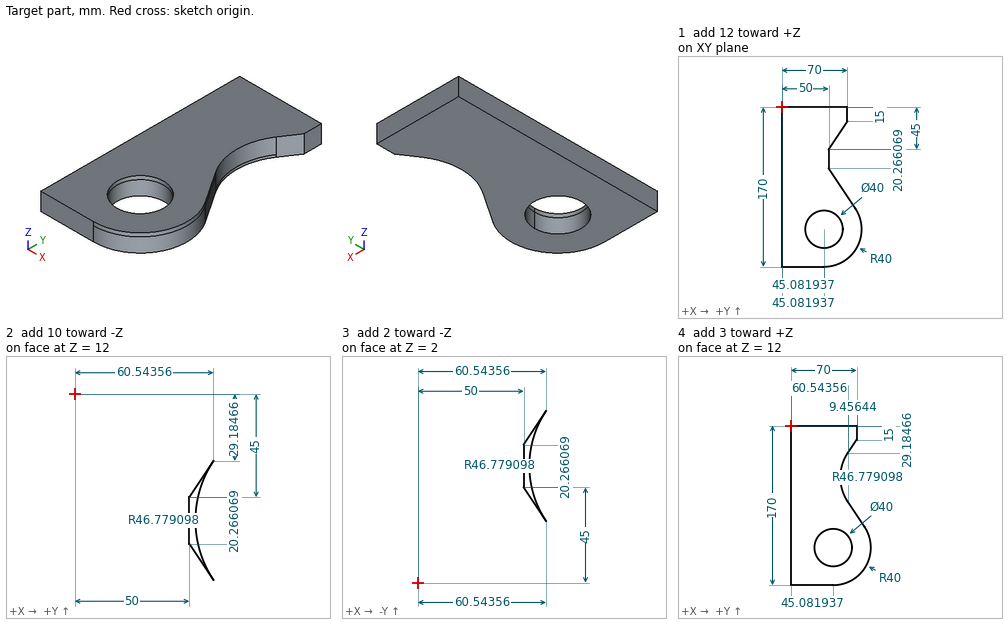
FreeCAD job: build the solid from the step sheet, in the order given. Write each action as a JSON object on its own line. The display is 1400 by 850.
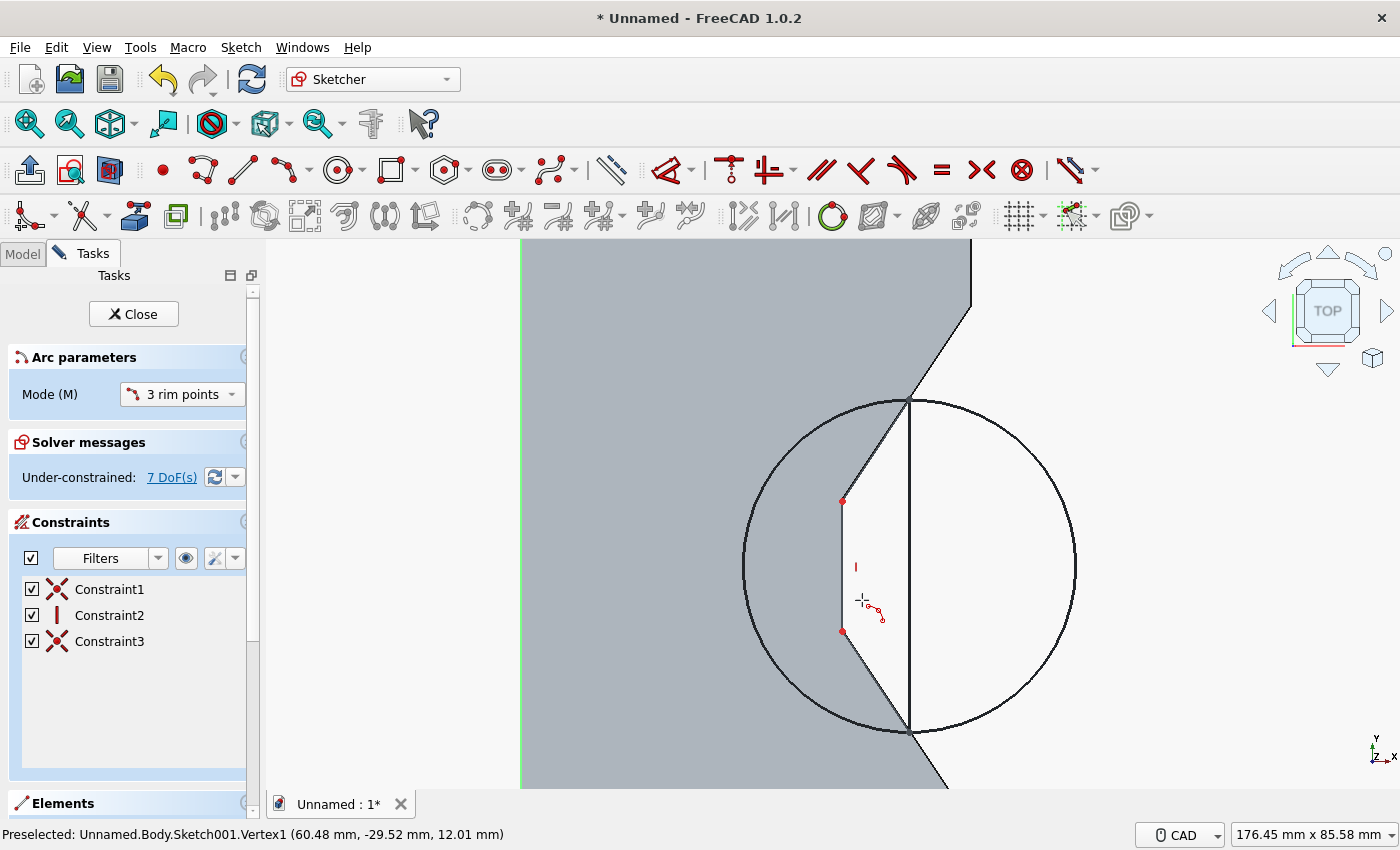
{"action": "left_click", "coordinate": [861, 600]}
{"action": "key", "text": "Escape"}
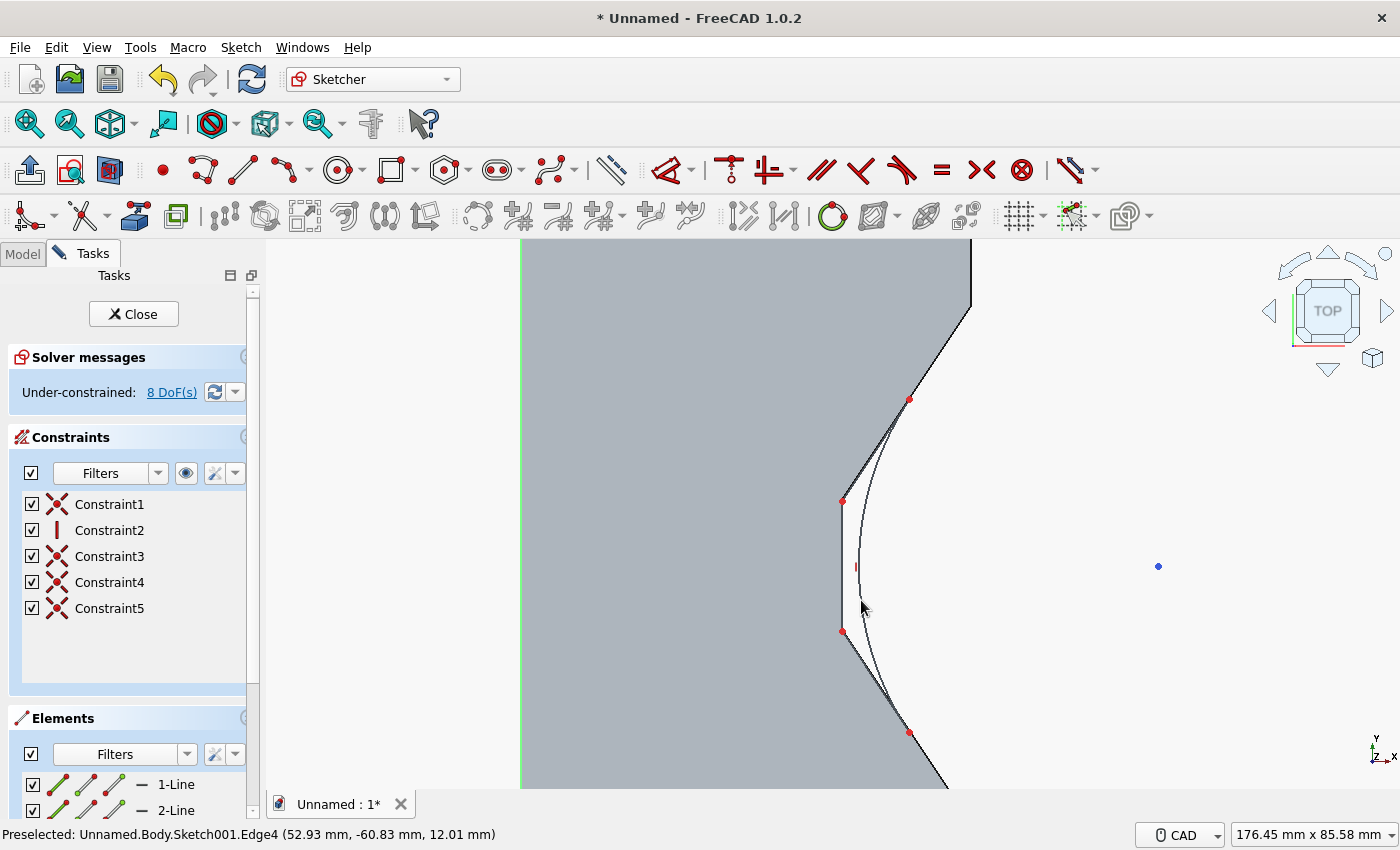
{"action": "left_click", "coordinate": [862, 471]}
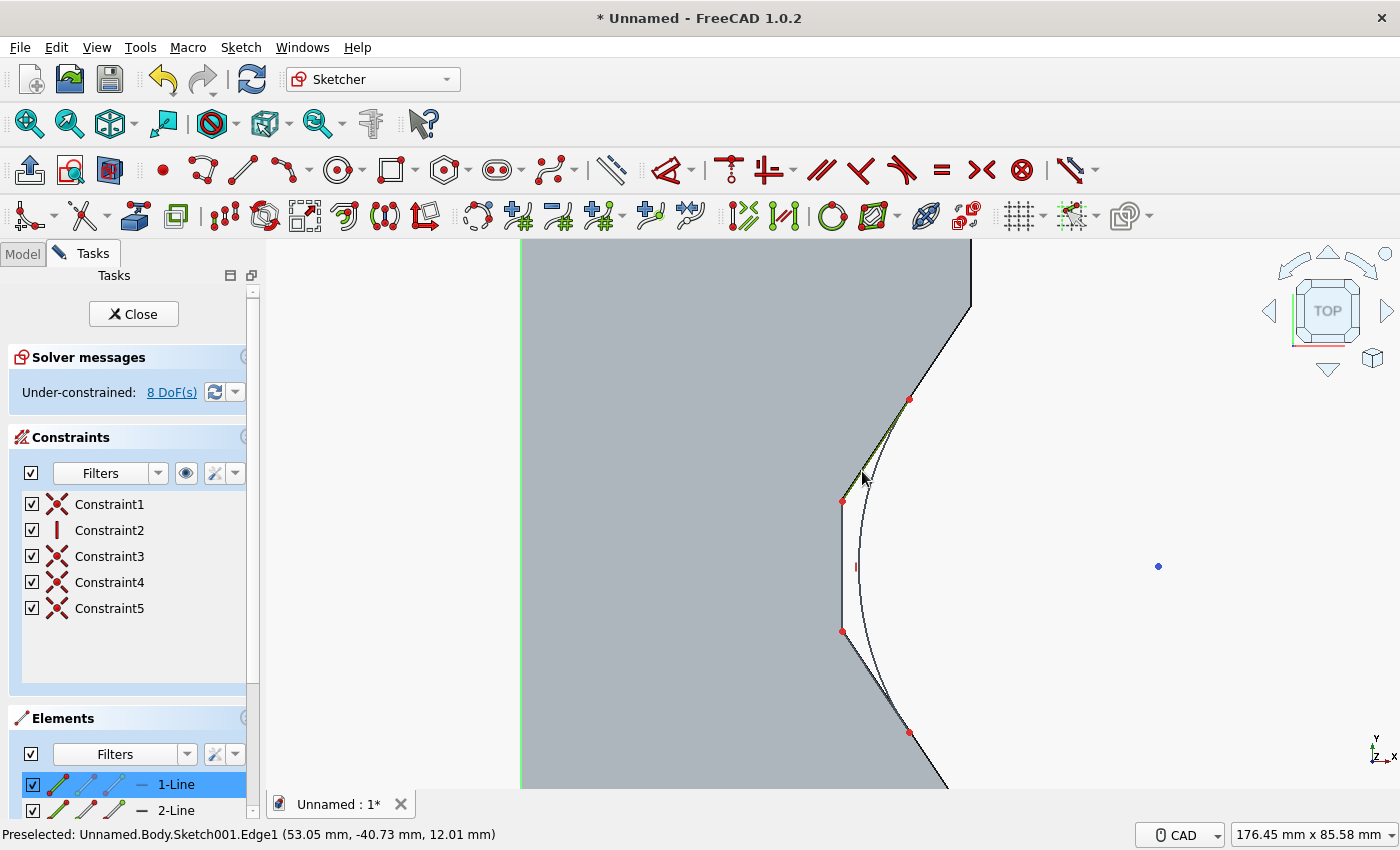
{"action": "left_click", "coordinate": [867, 496]}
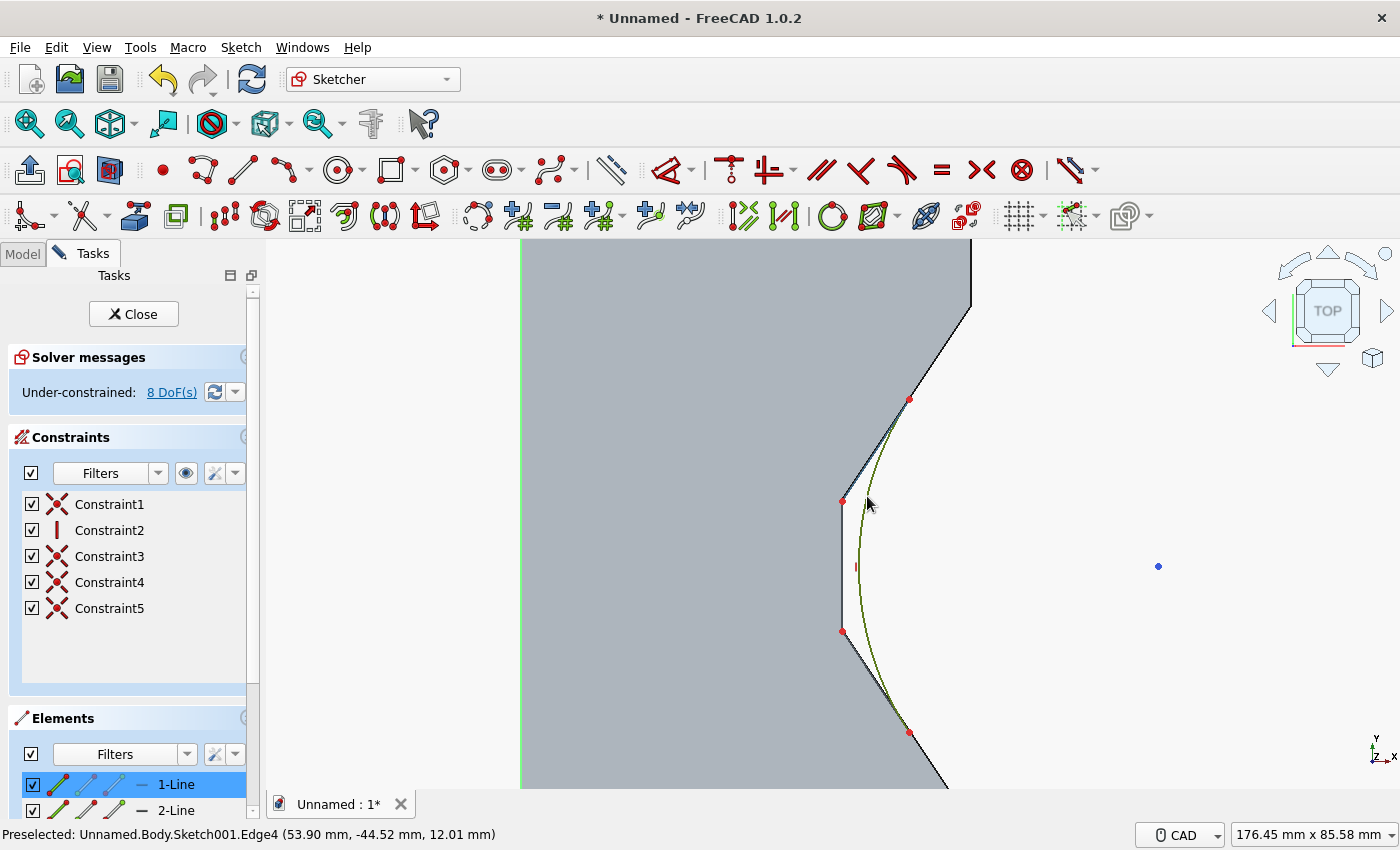
{"action": "left_click", "coordinate": [902, 170]}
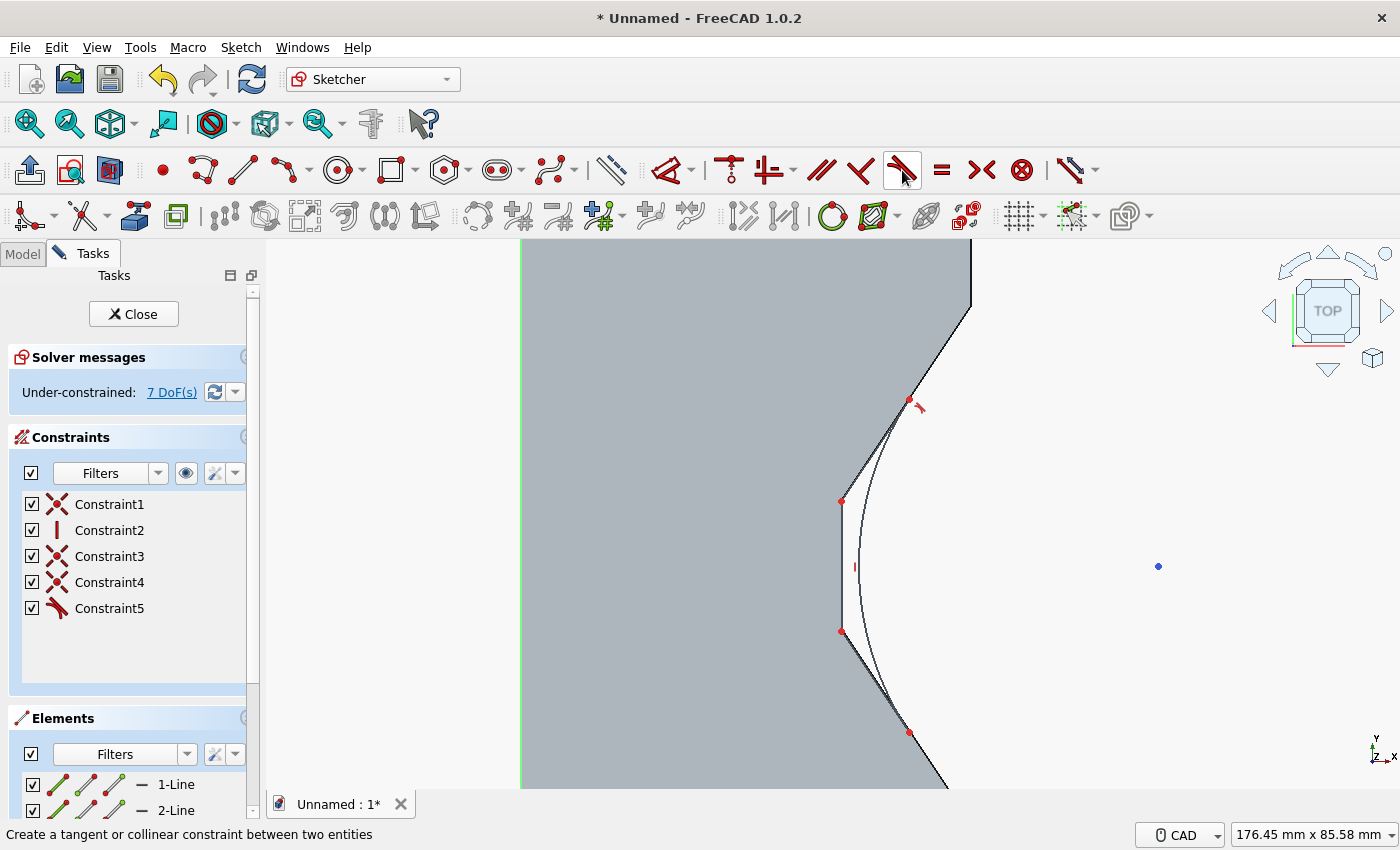
{"action": "left_click", "coordinate": [862, 661]}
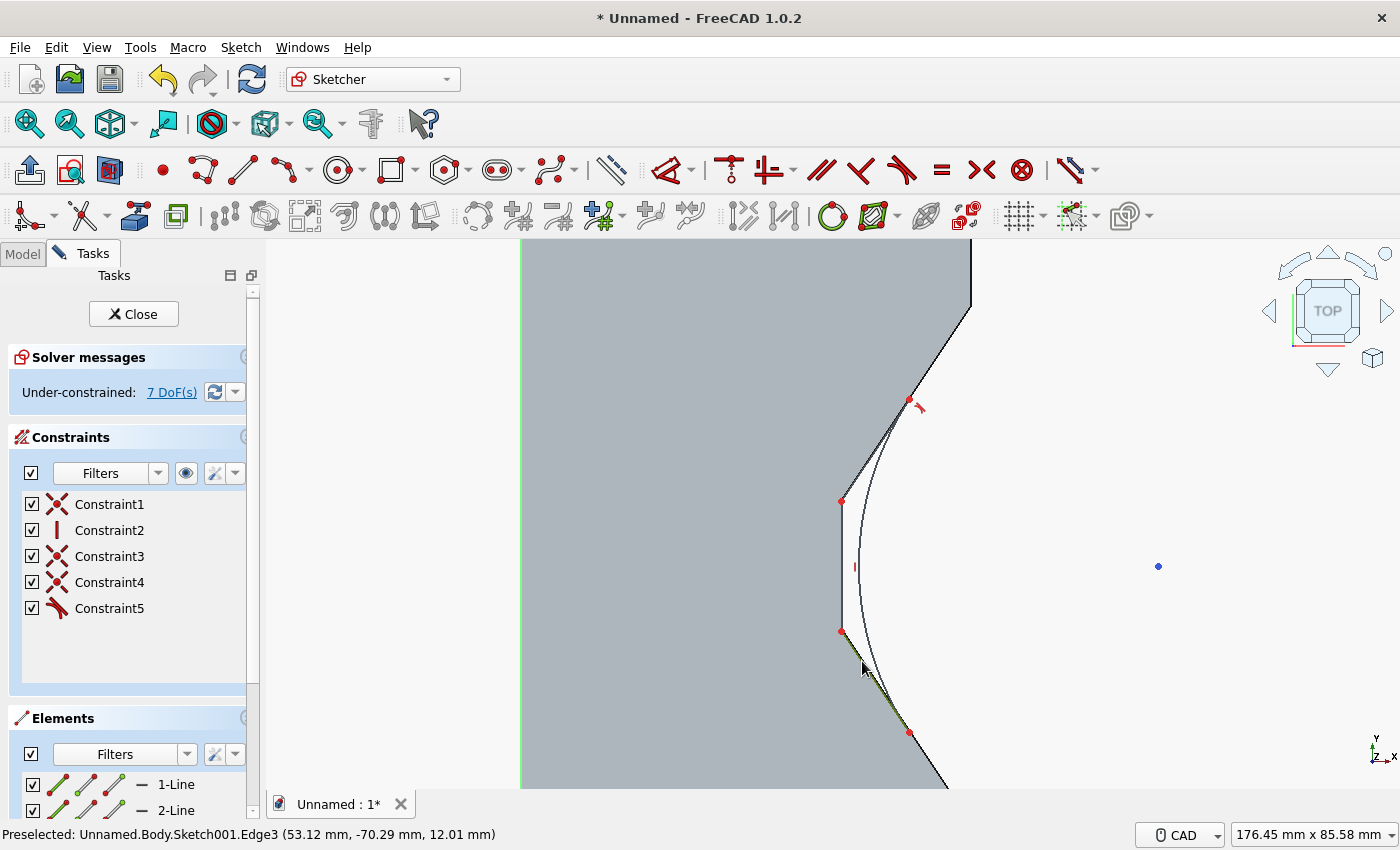
{"action": "left_click", "coordinate": [867, 496]}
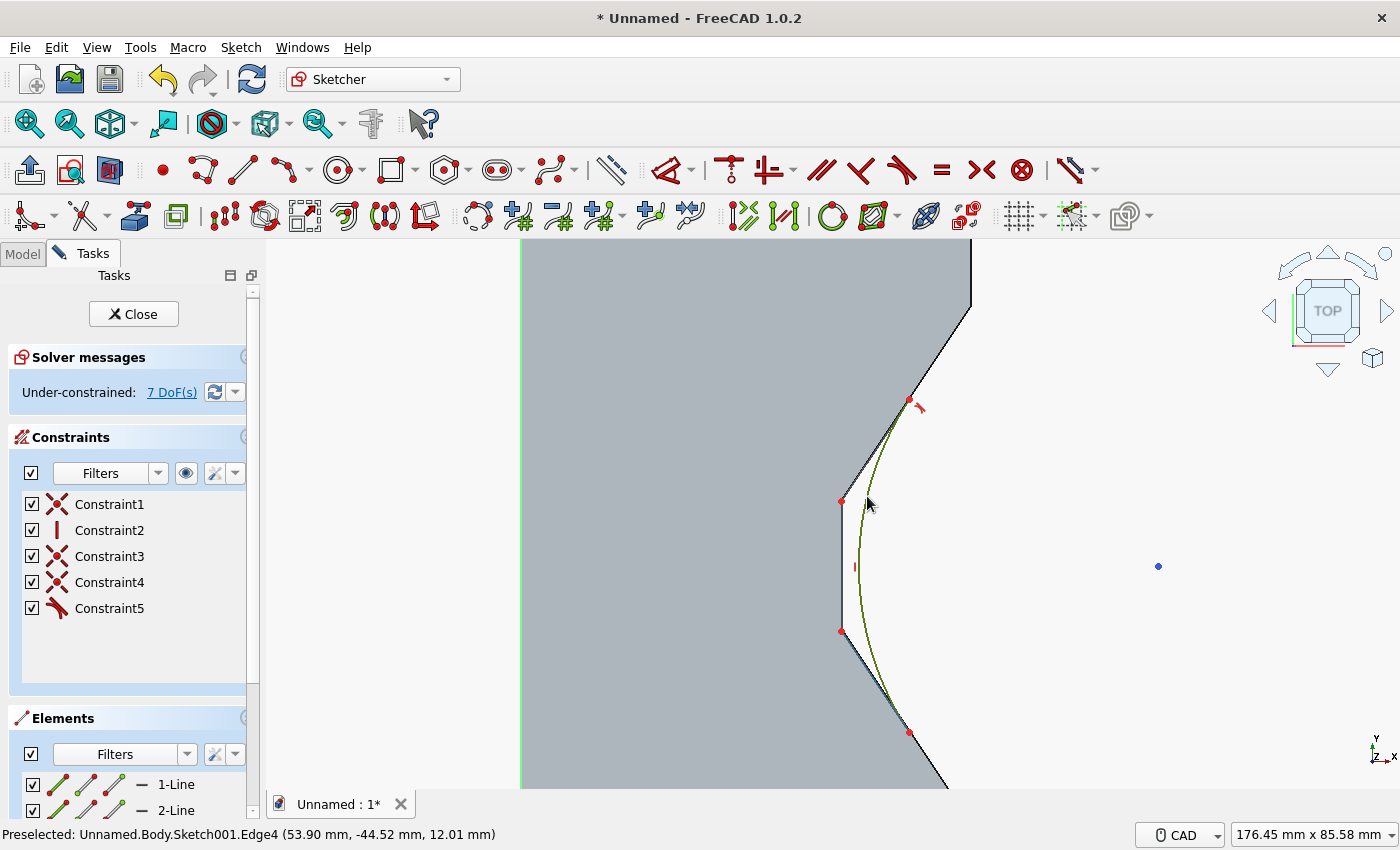
{"action": "left_click", "coordinate": [902, 170]}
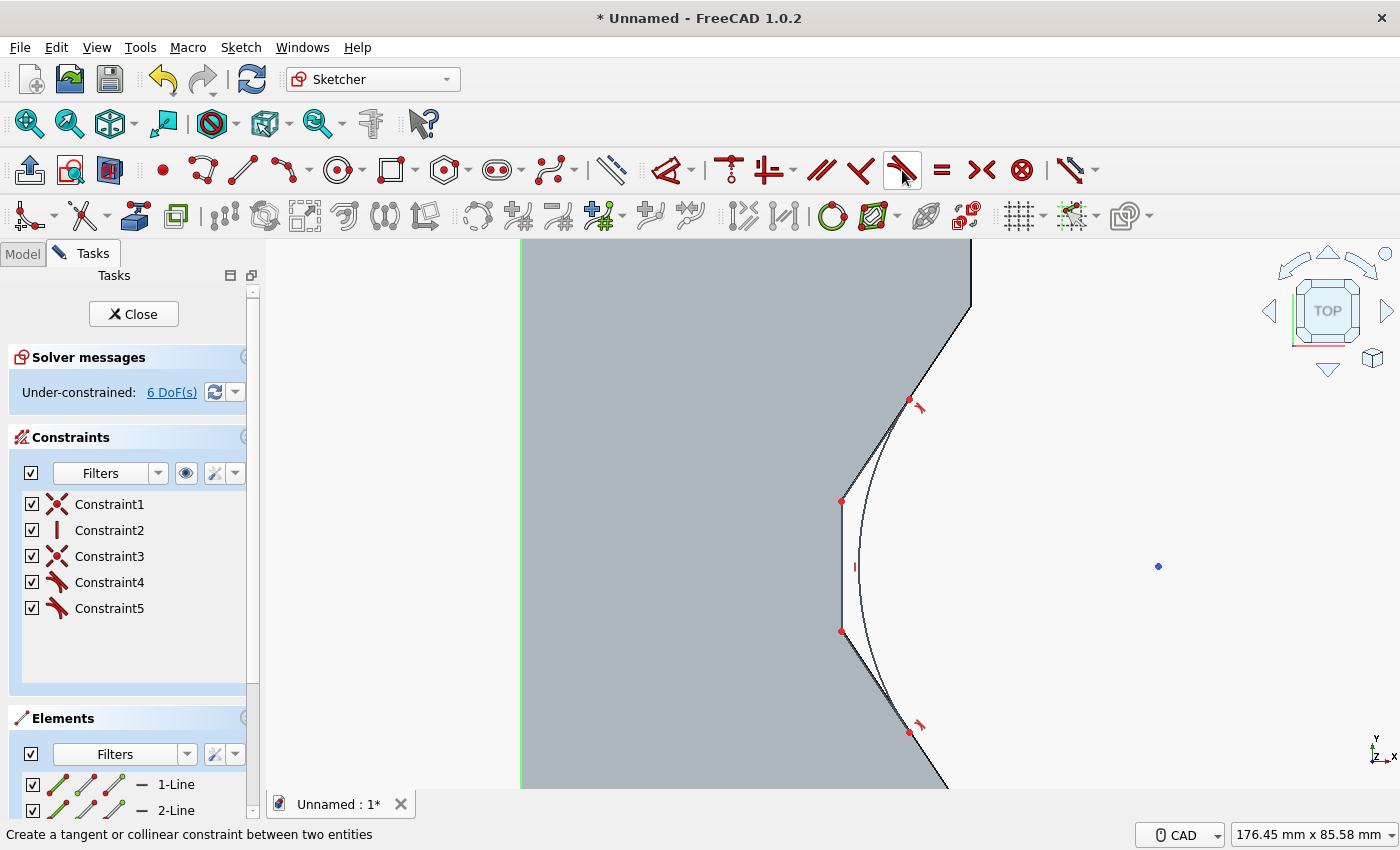
{"action": "left_click", "coordinate": [666, 170]}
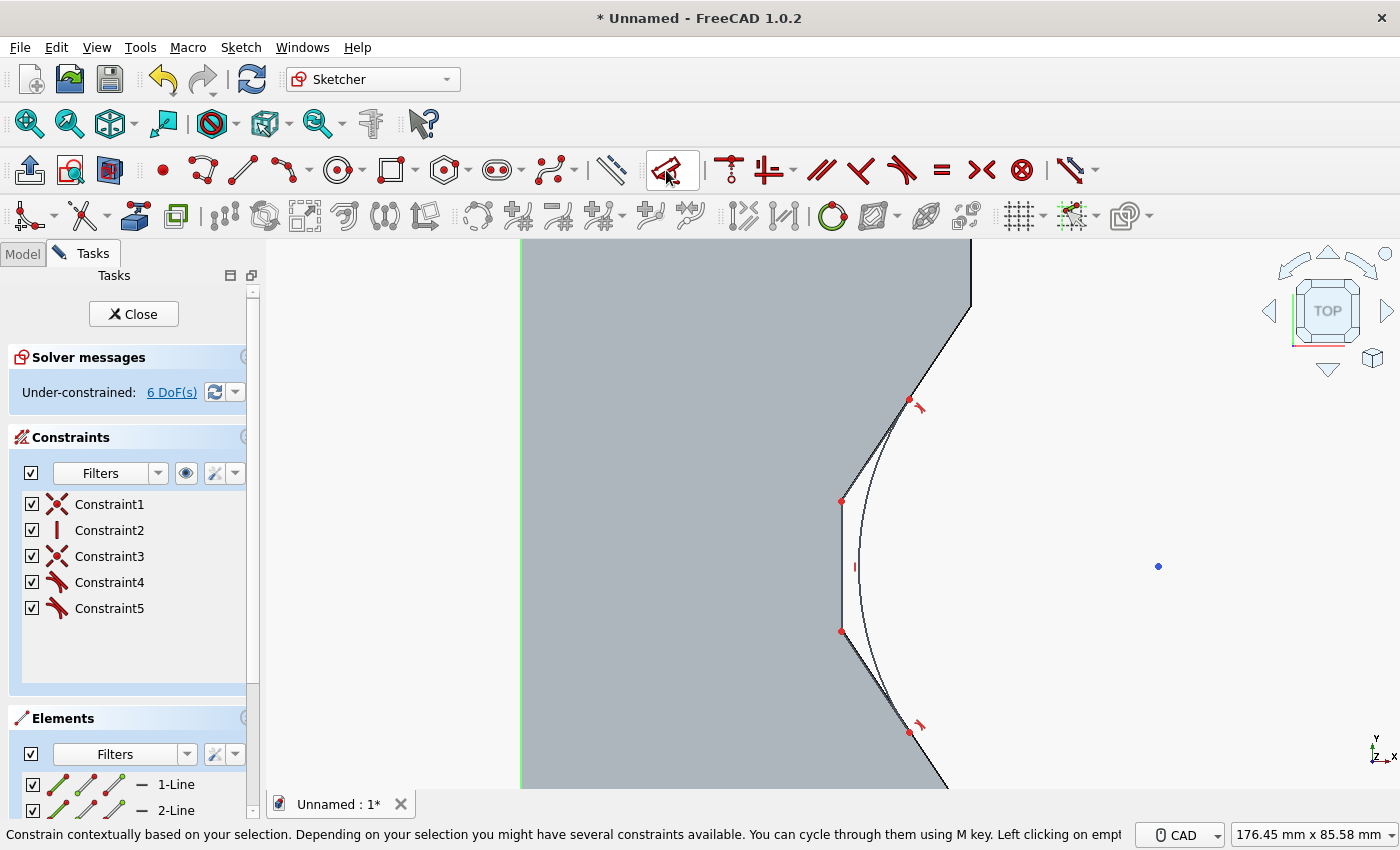
{"action": "left_click", "coordinate": [867, 496]}
{"action": "left_click", "coordinate": [913, 344]}